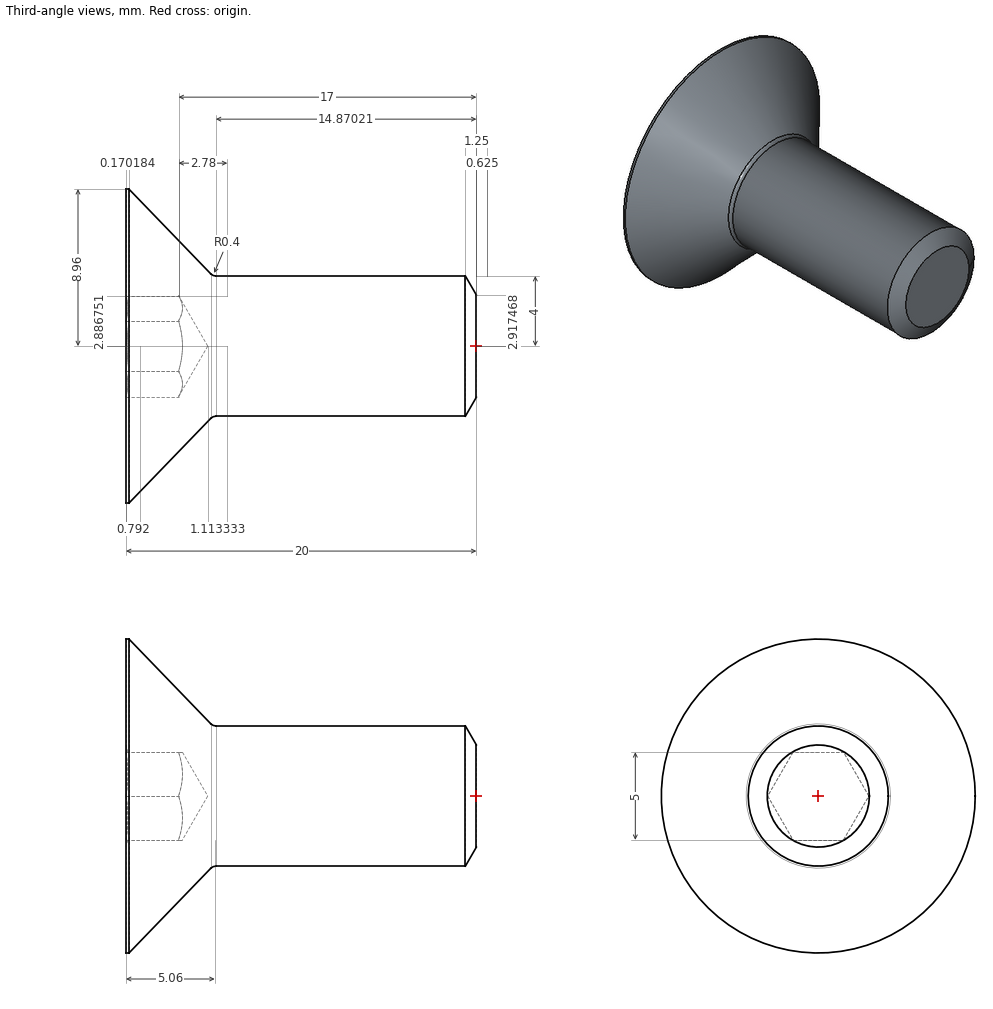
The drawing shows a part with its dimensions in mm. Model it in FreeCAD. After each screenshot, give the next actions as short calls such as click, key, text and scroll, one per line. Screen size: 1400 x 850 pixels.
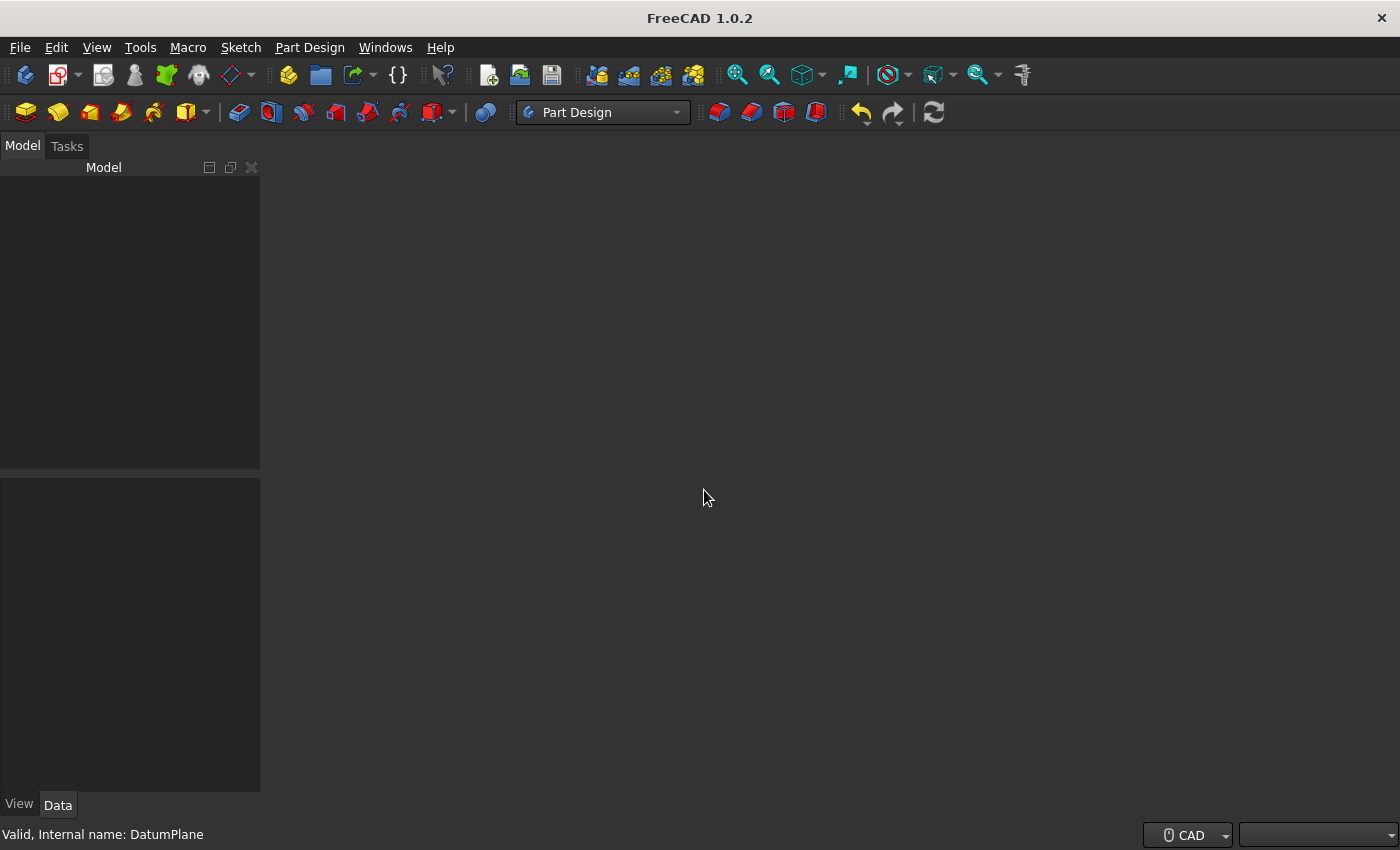
click(488, 76)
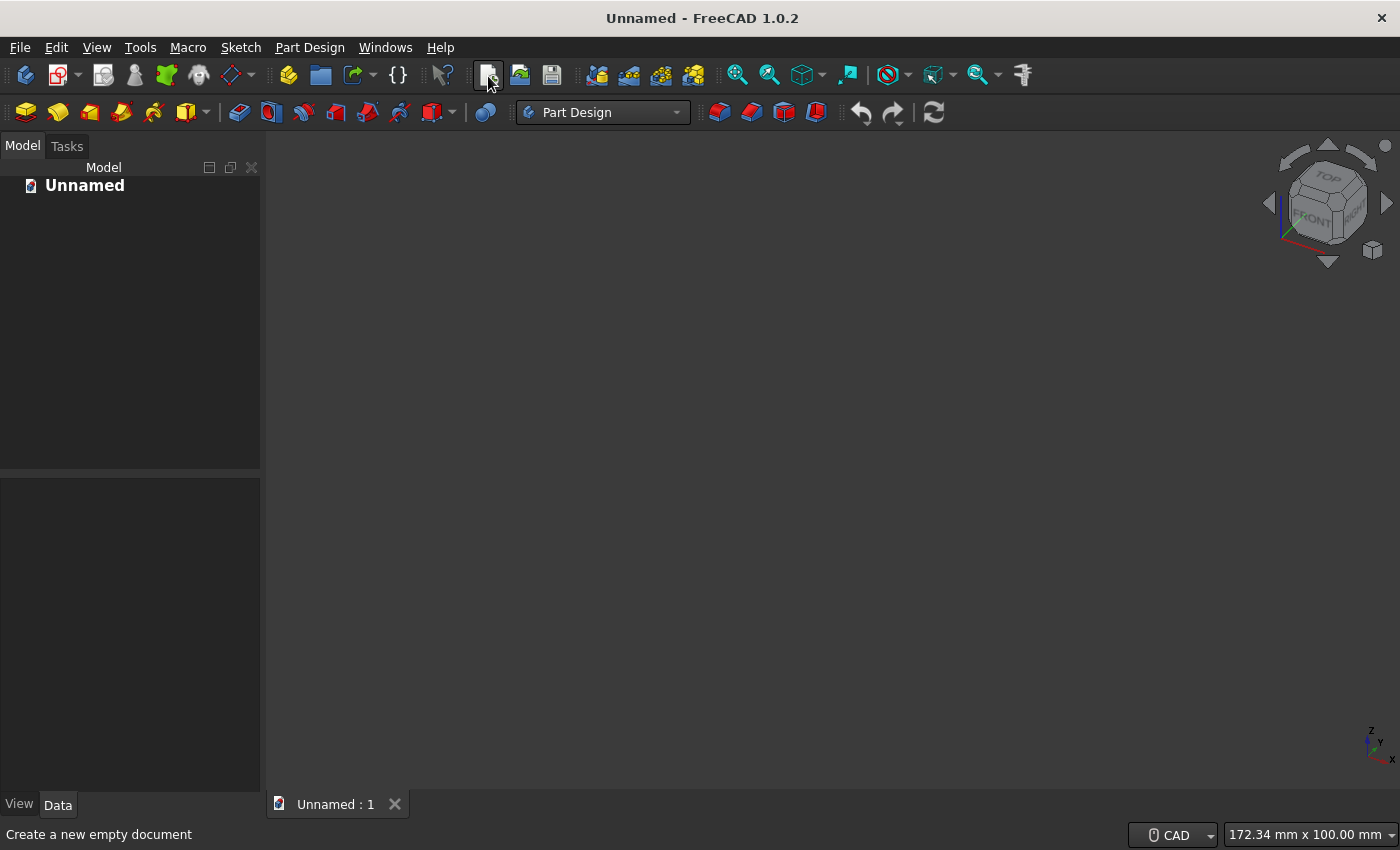
click(58, 76)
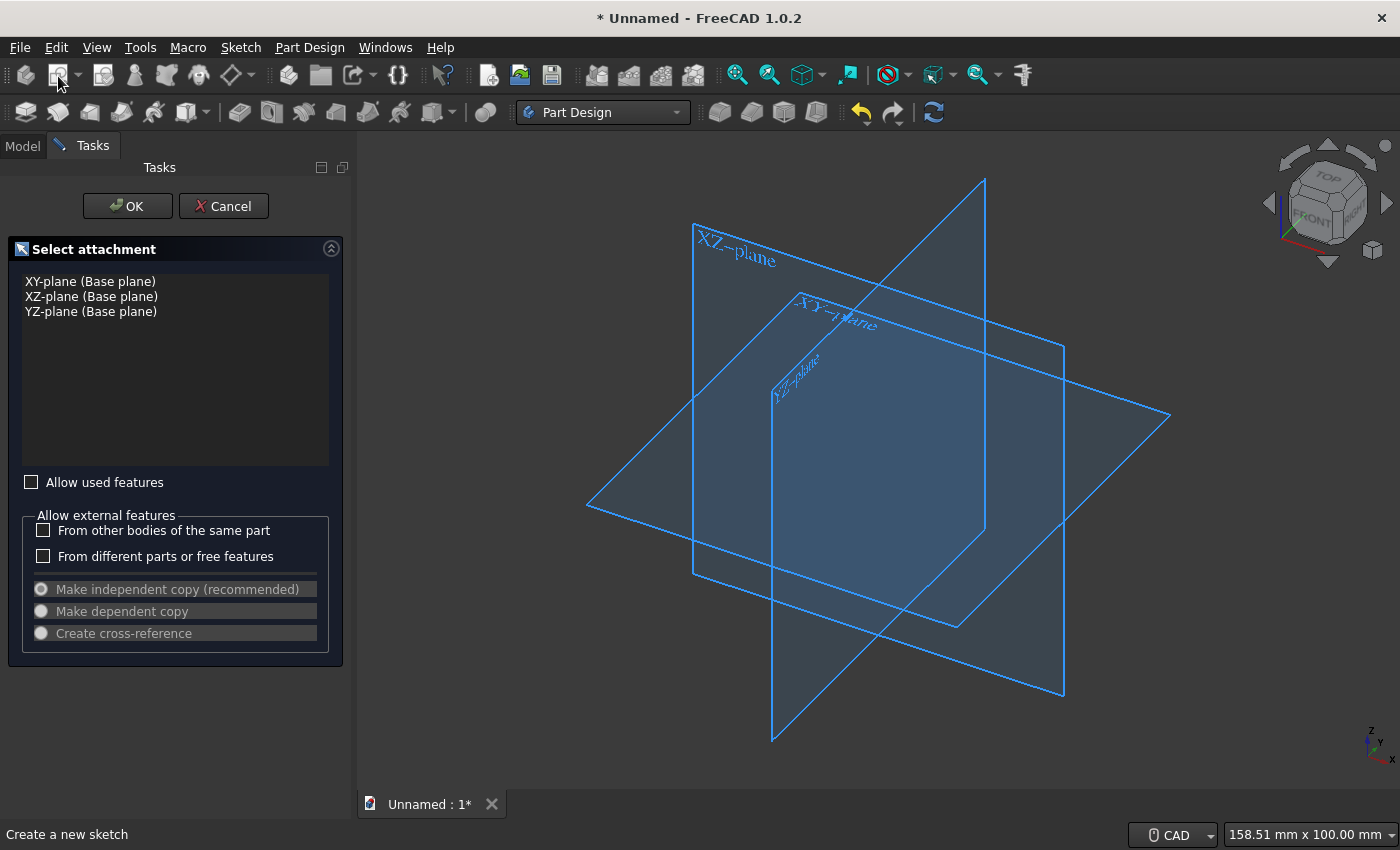
click(82, 282)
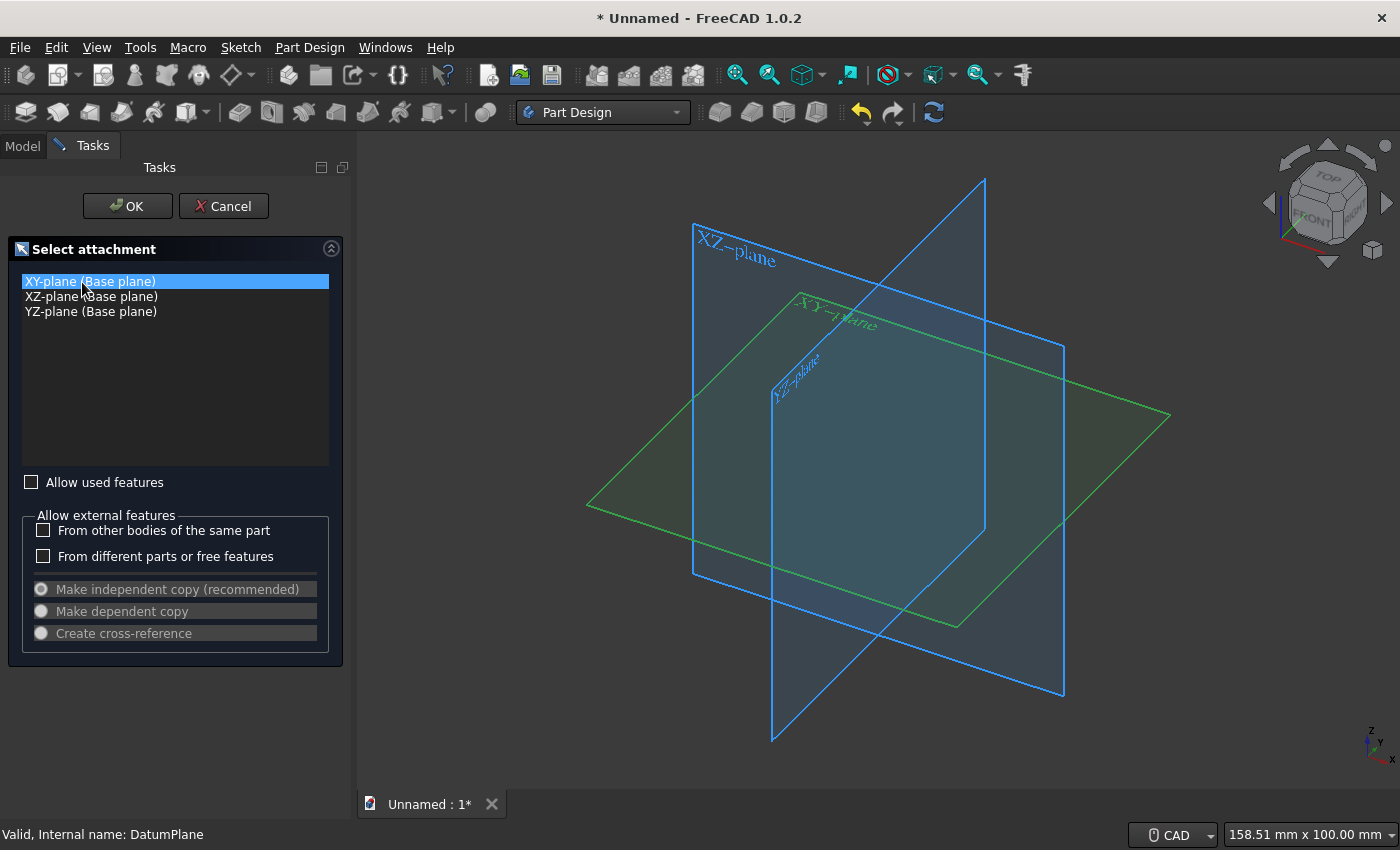
click(128, 206)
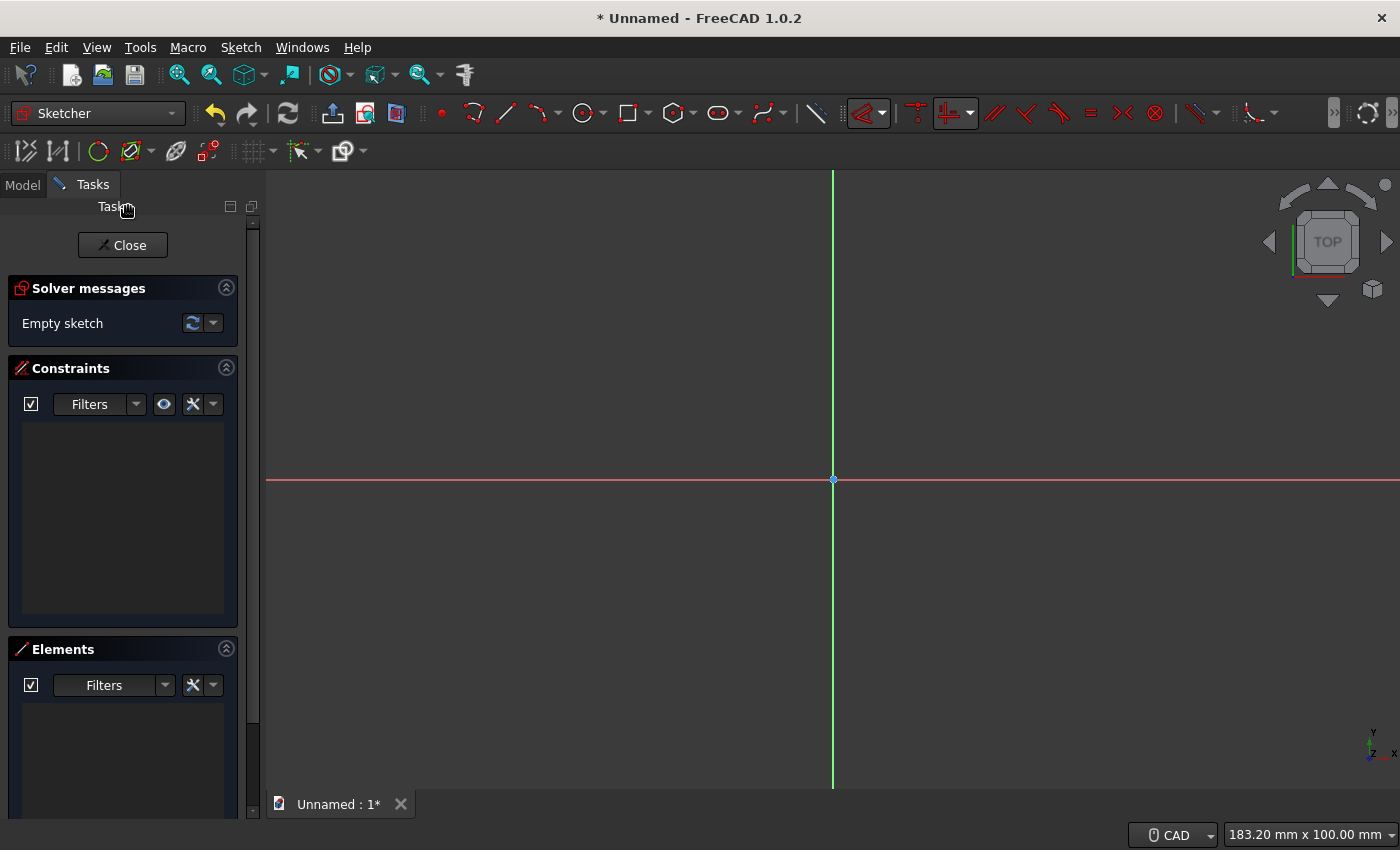
scroll(773, 445, up, 8)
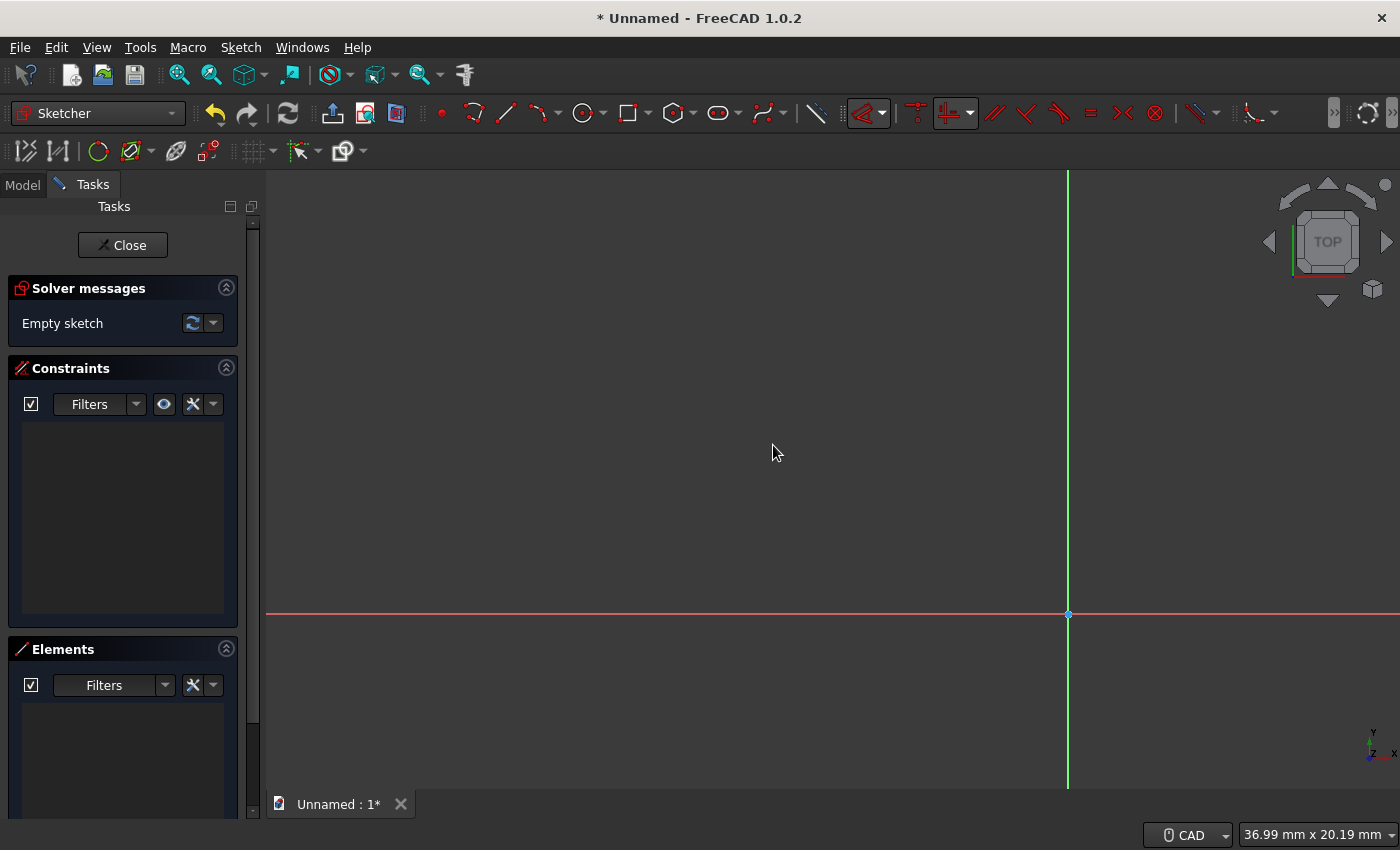
click(474, 114)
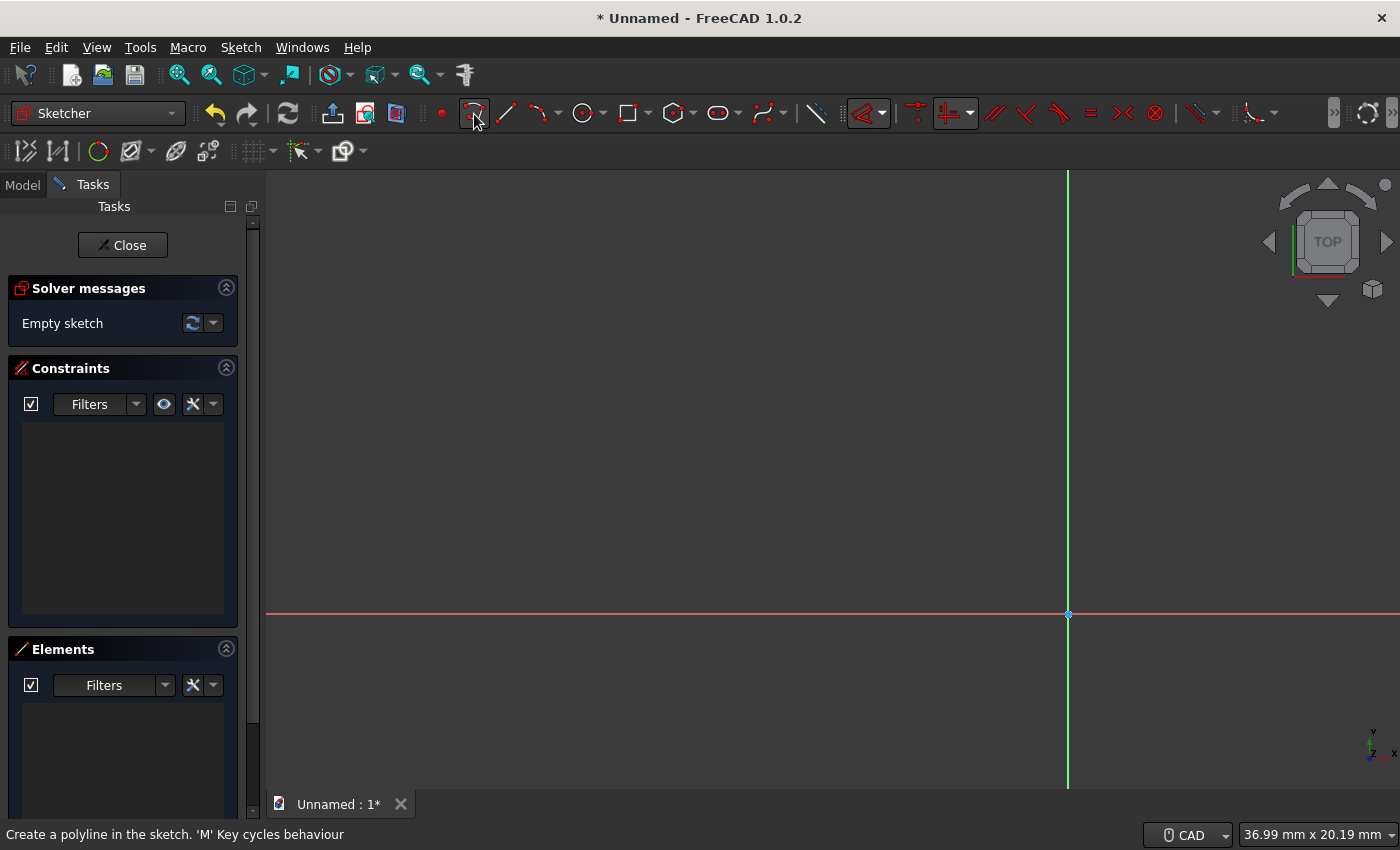
click(604, 488)
click(460, 339)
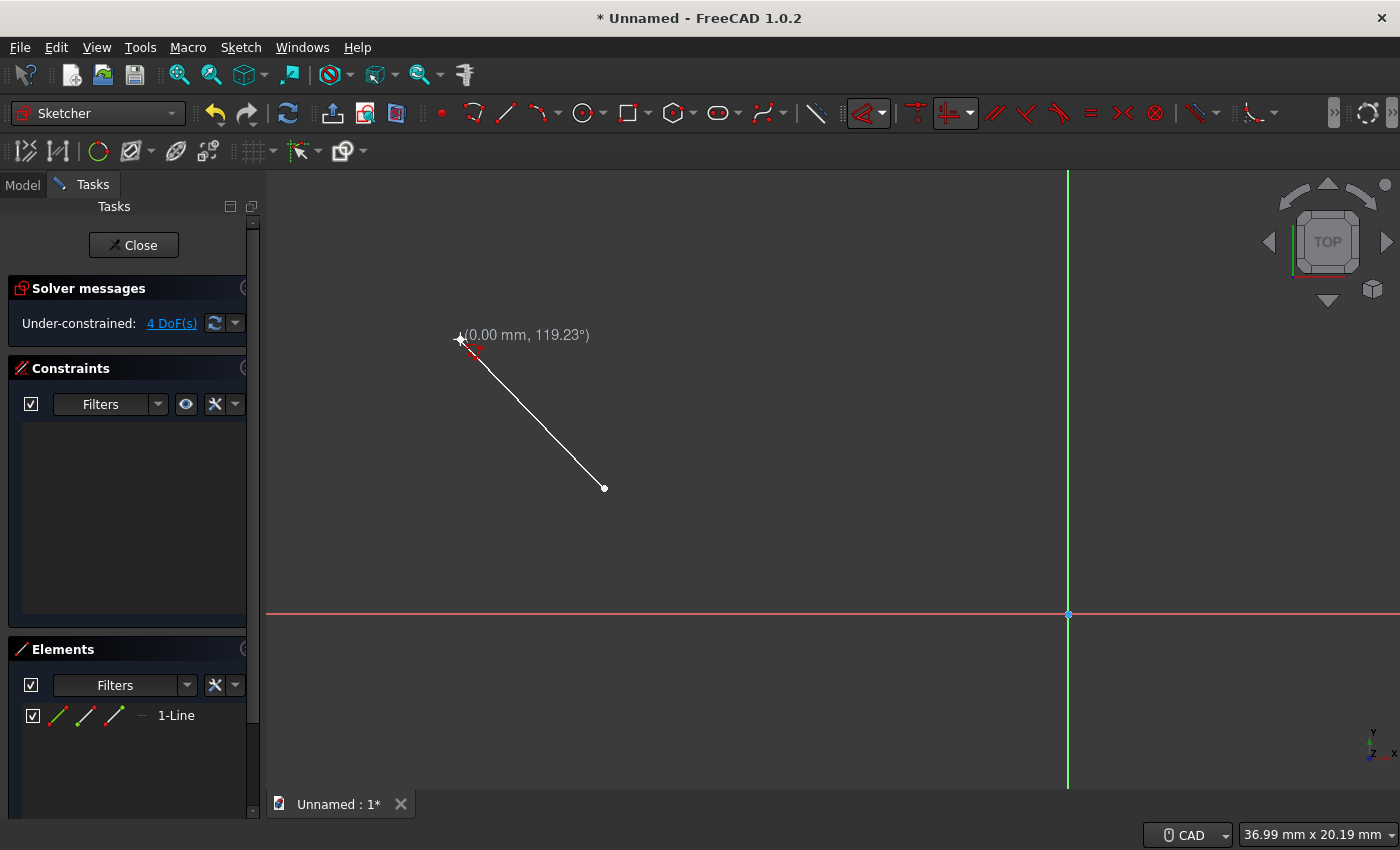
scroll(455, 339, up, 6)